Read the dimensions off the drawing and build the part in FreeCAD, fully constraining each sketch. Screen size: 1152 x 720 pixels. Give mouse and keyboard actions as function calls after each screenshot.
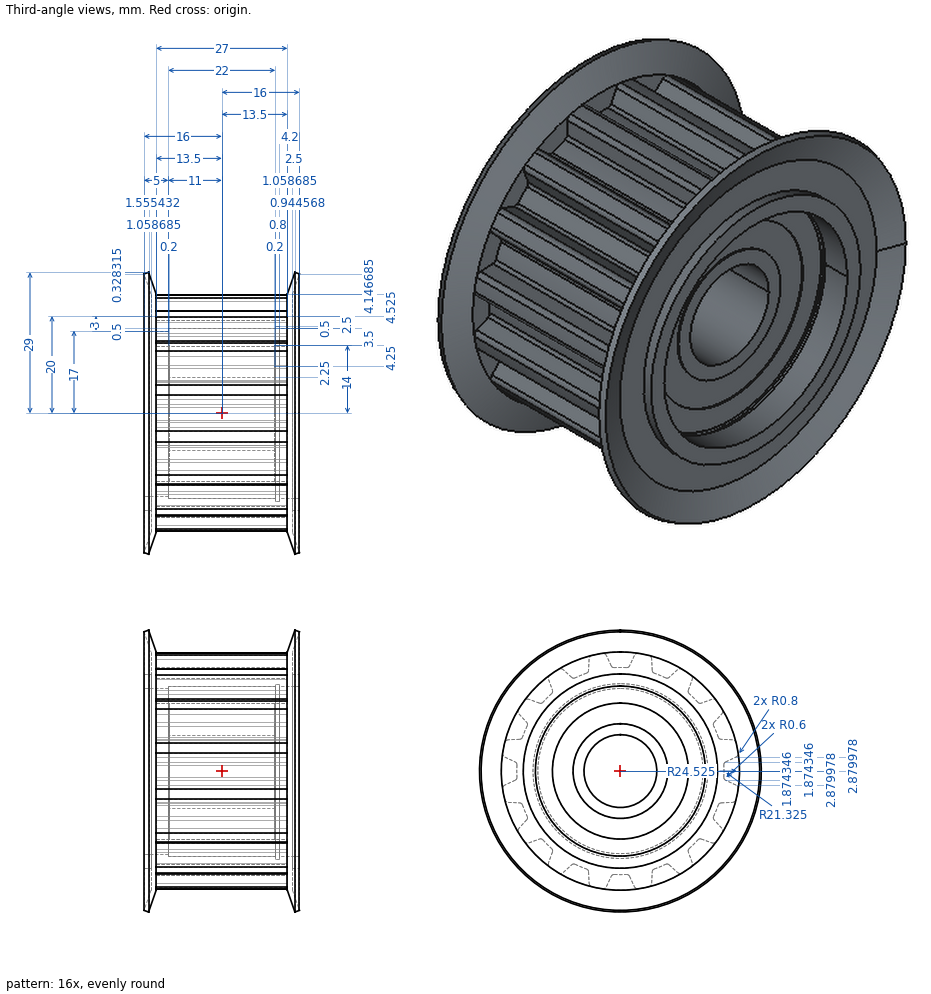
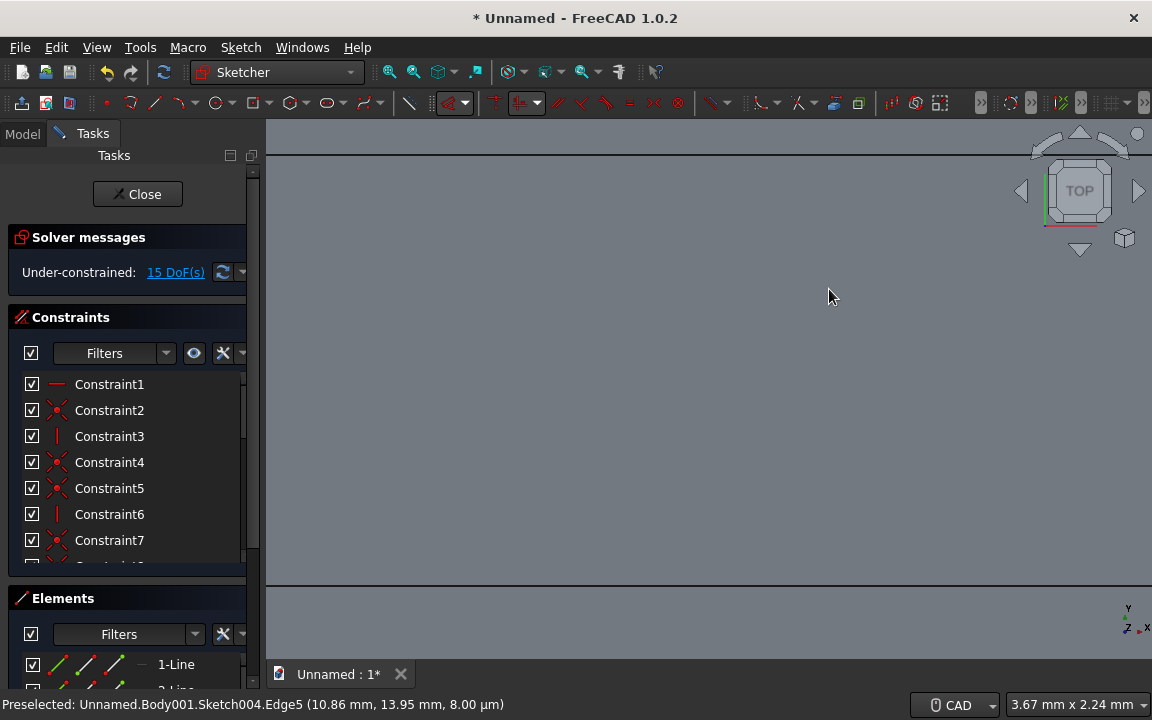
key(h)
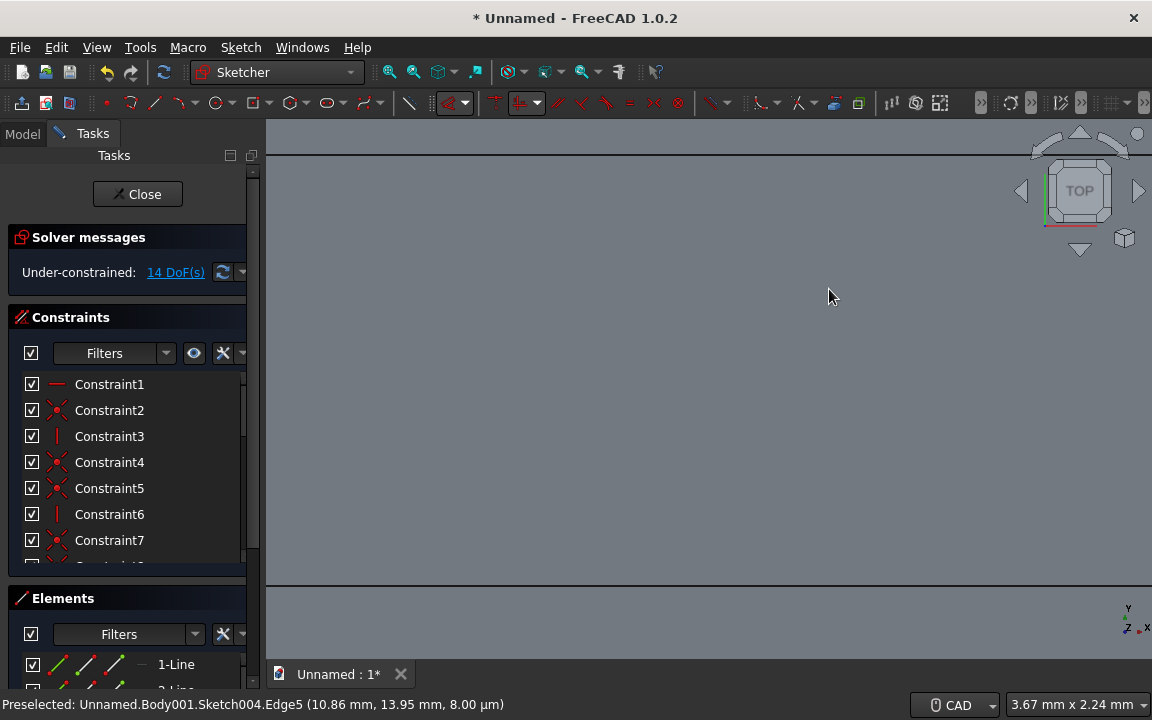
scroll(836, 296, down, 13)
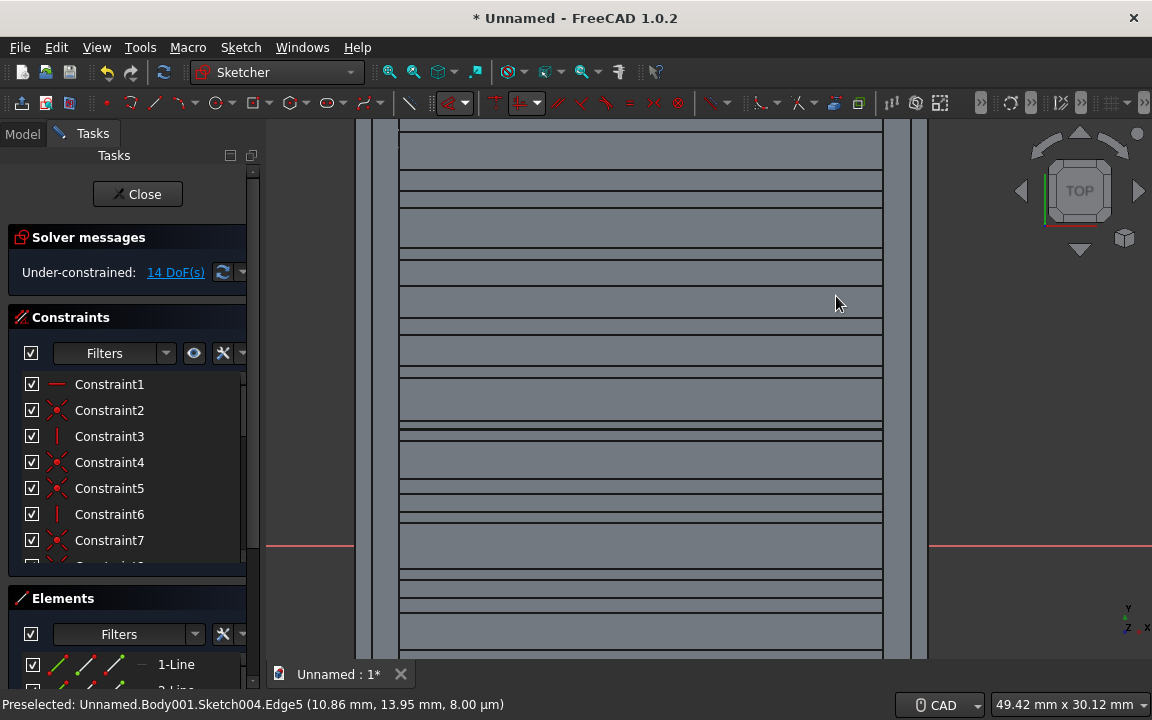
scroll(445, 296, up, 13)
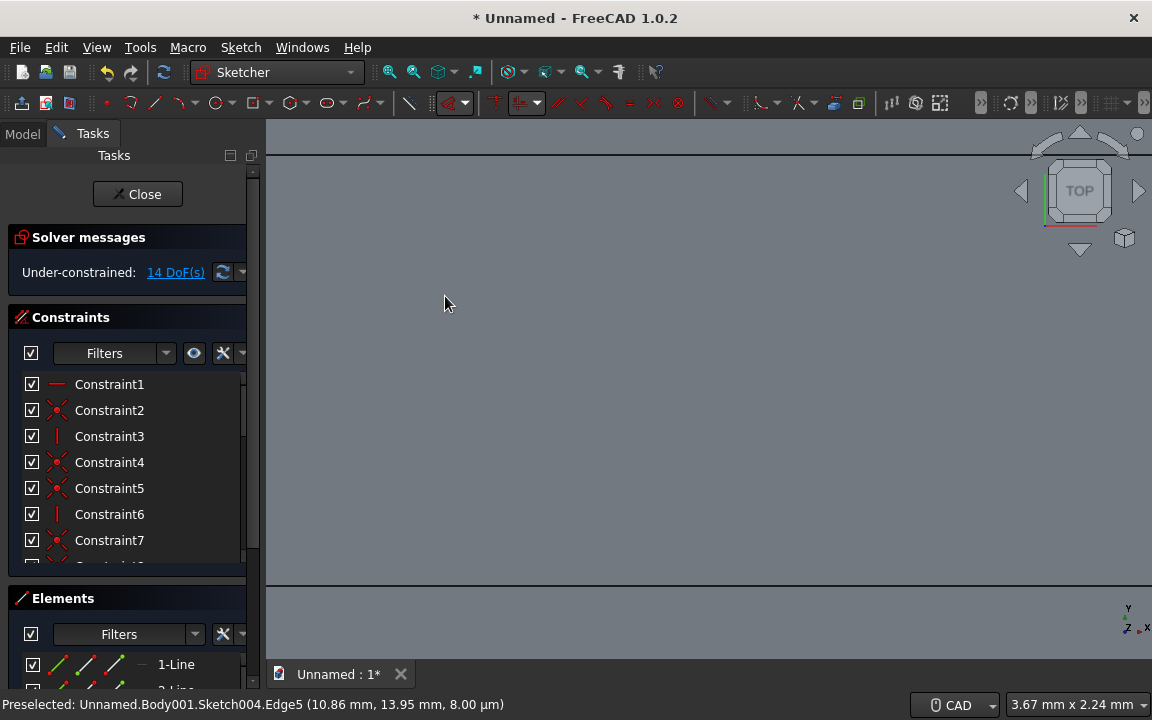
click(445, 289)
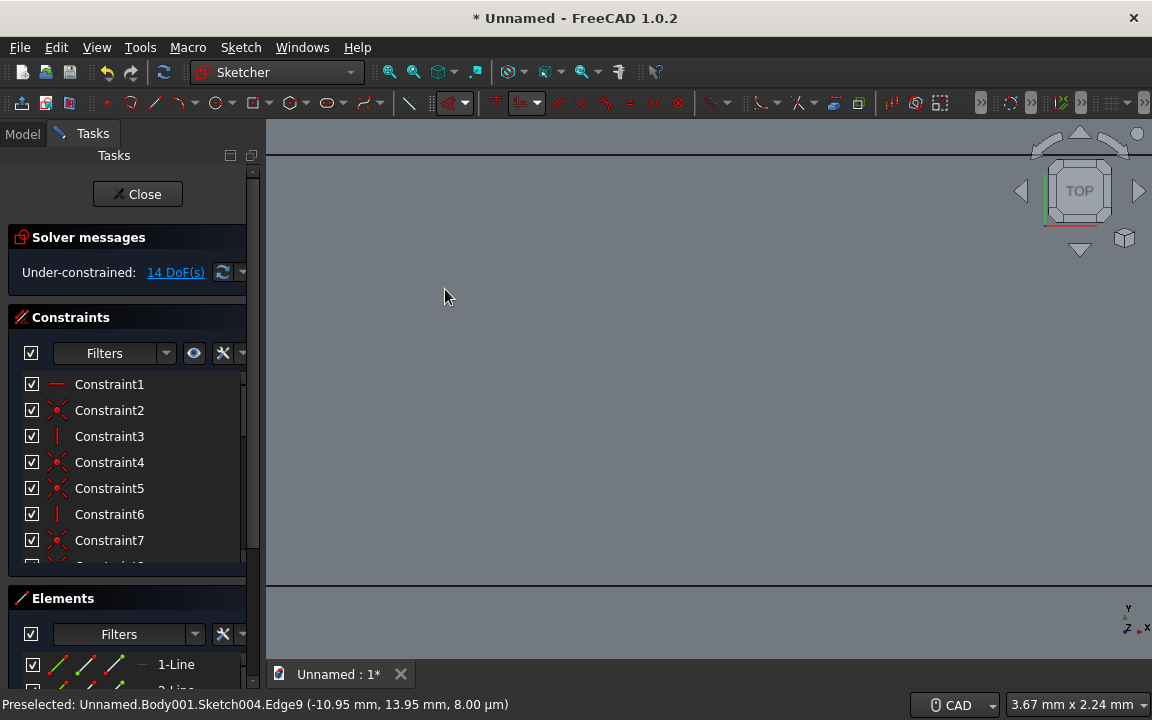
key(h)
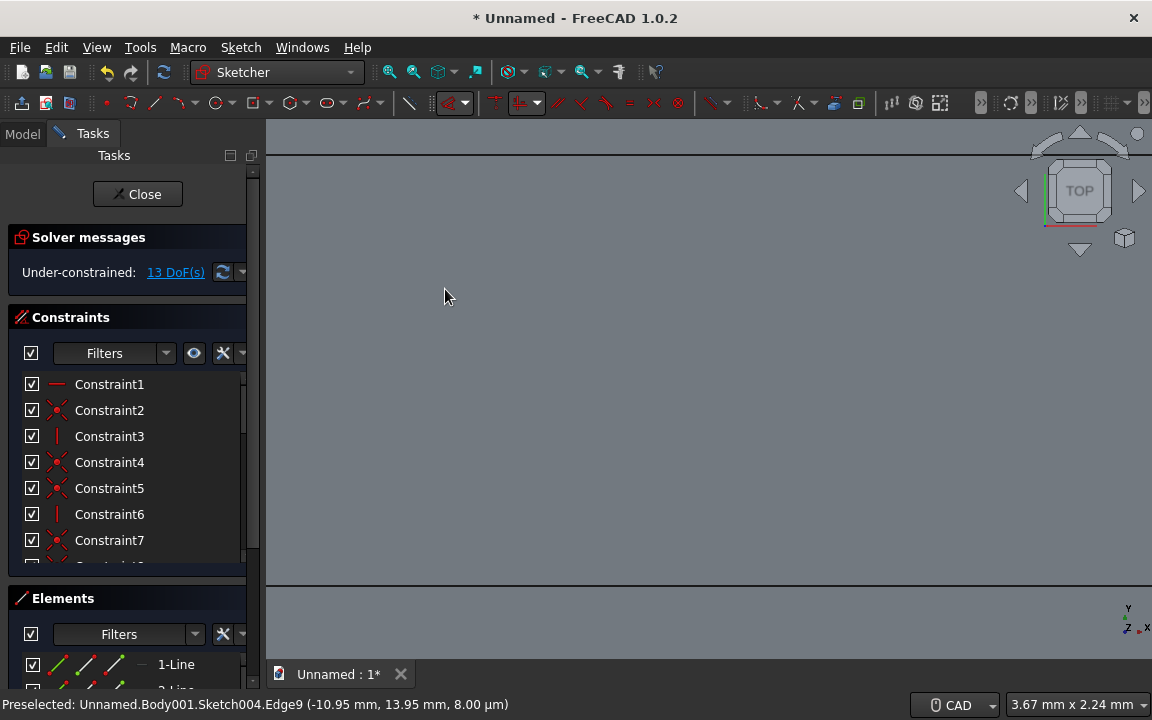
scroll(444, 296, down, 13)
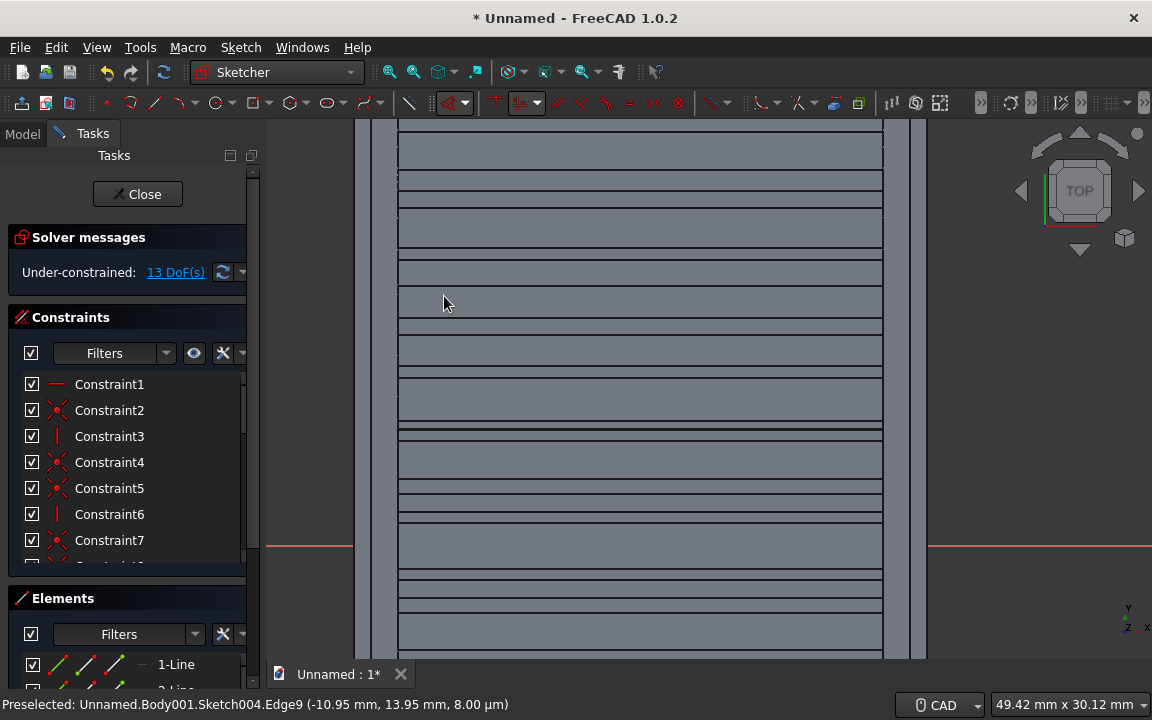
scroll(446, 372, up, 13)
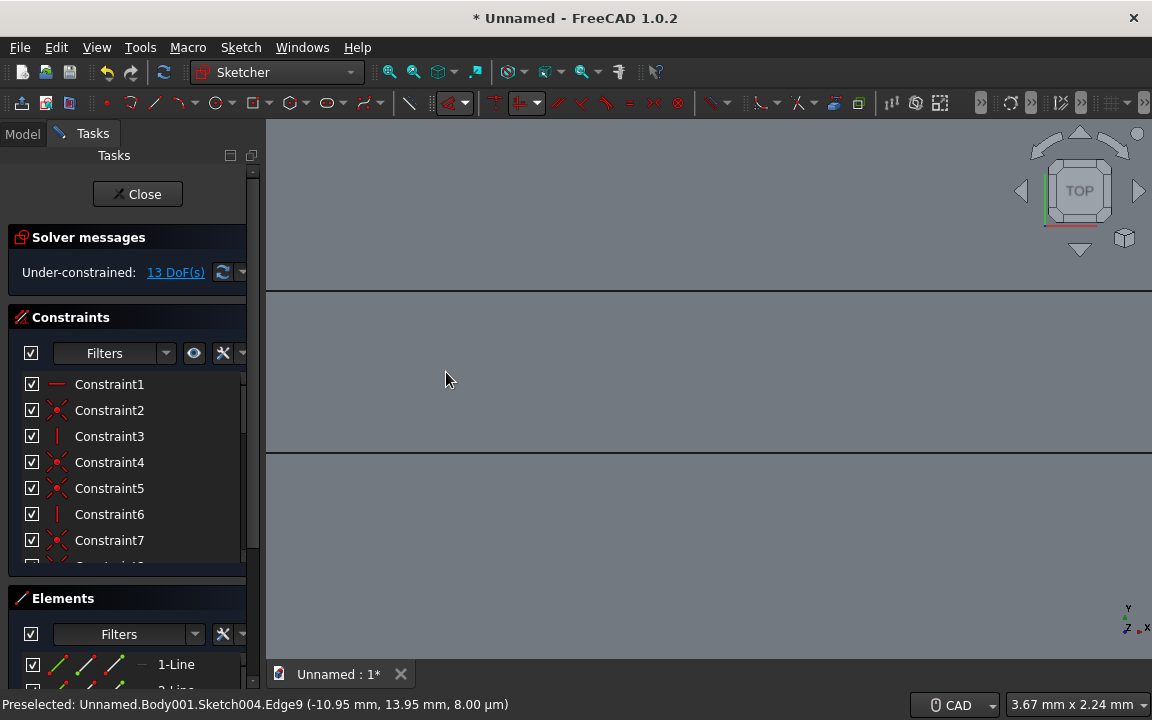
click(441, 363)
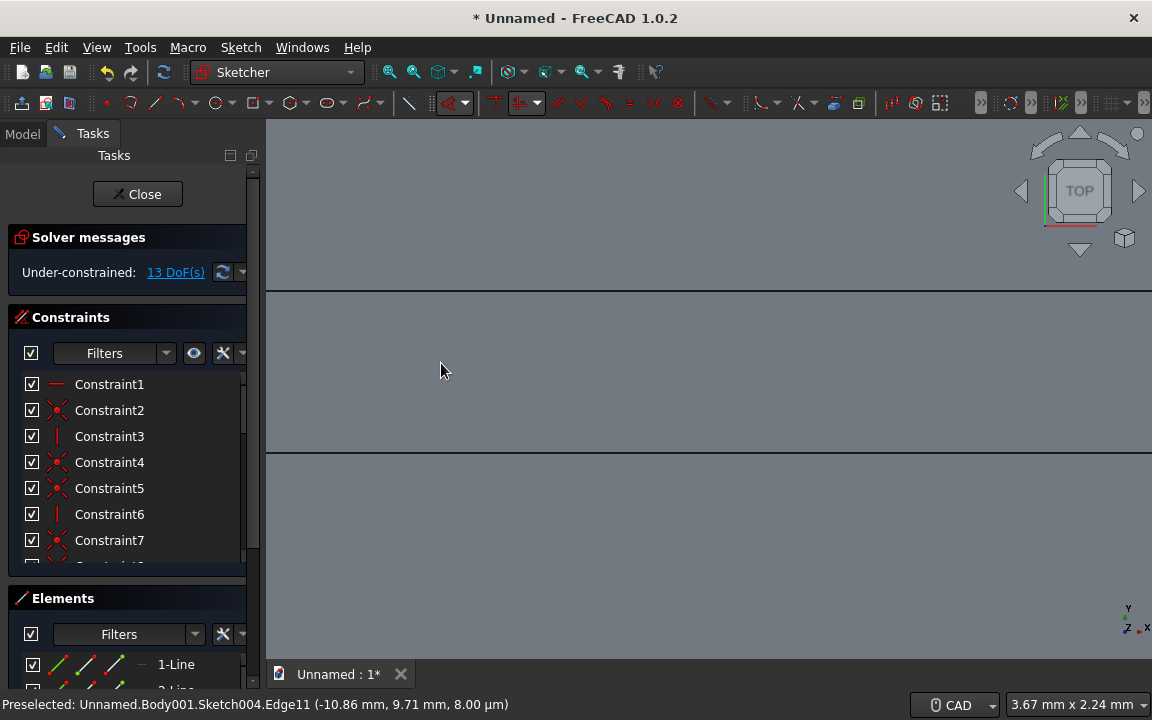
key(h)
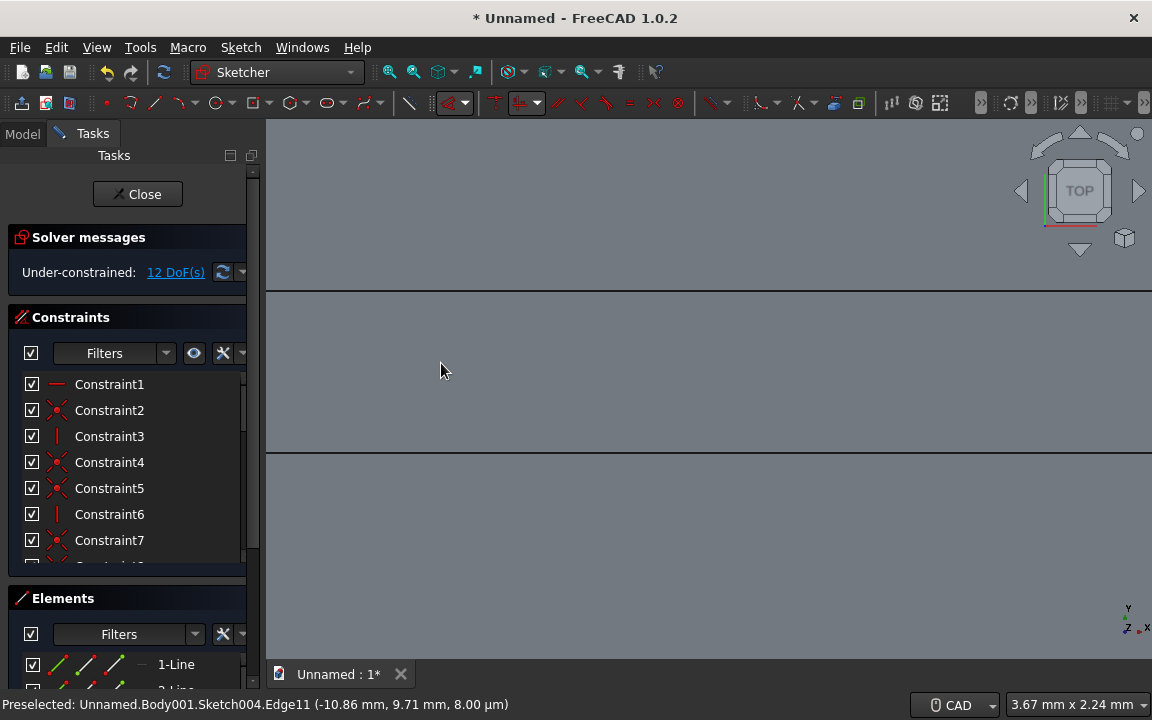
scroll(446, 372, down, 13)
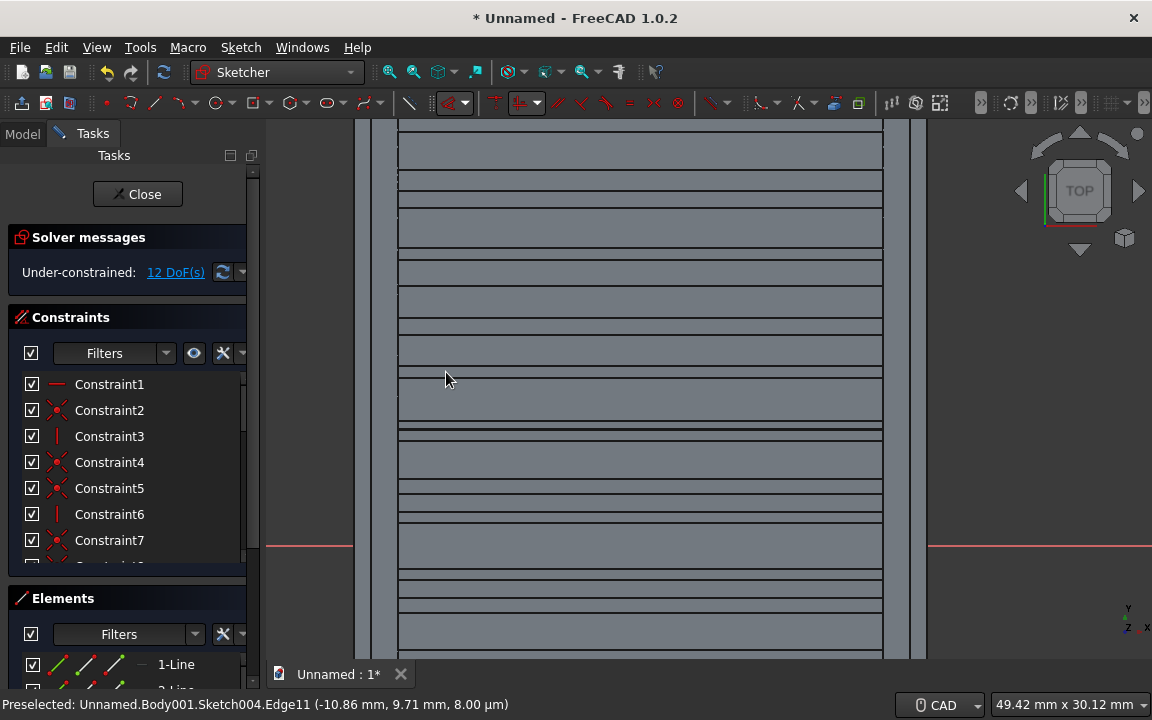
click(562, 412)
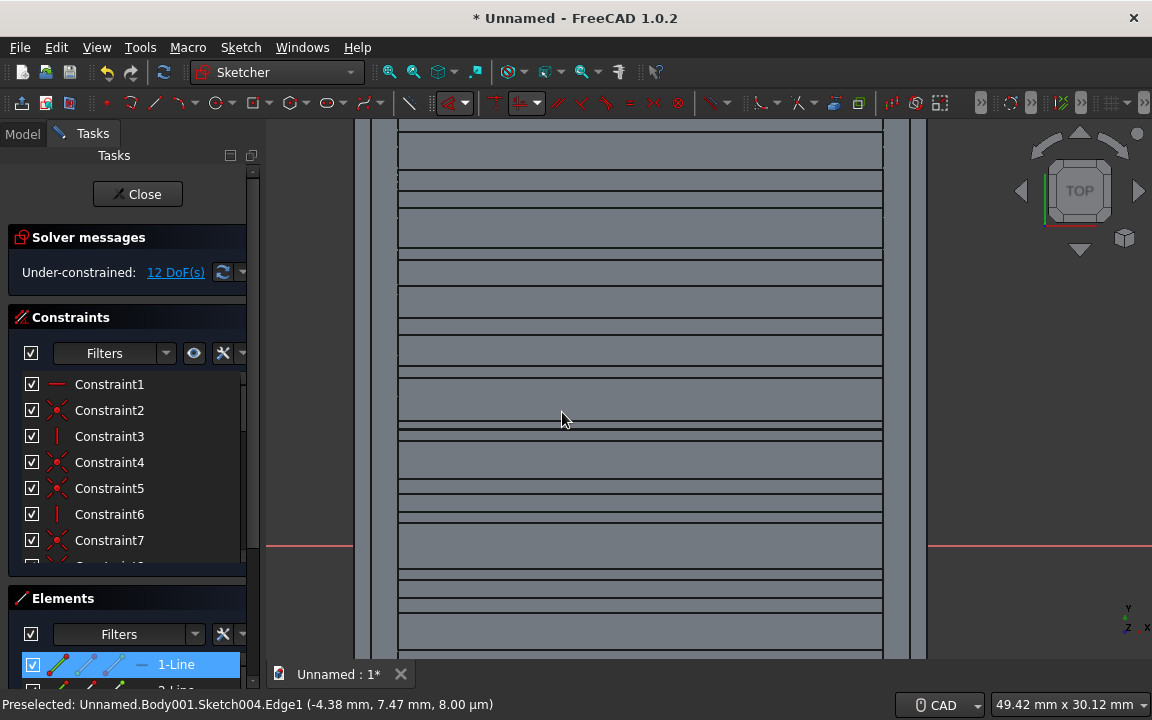
click(468, 104)